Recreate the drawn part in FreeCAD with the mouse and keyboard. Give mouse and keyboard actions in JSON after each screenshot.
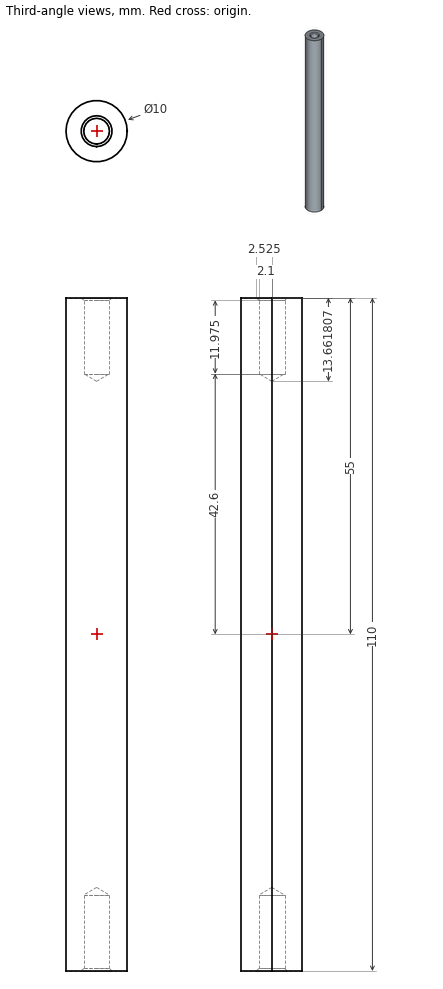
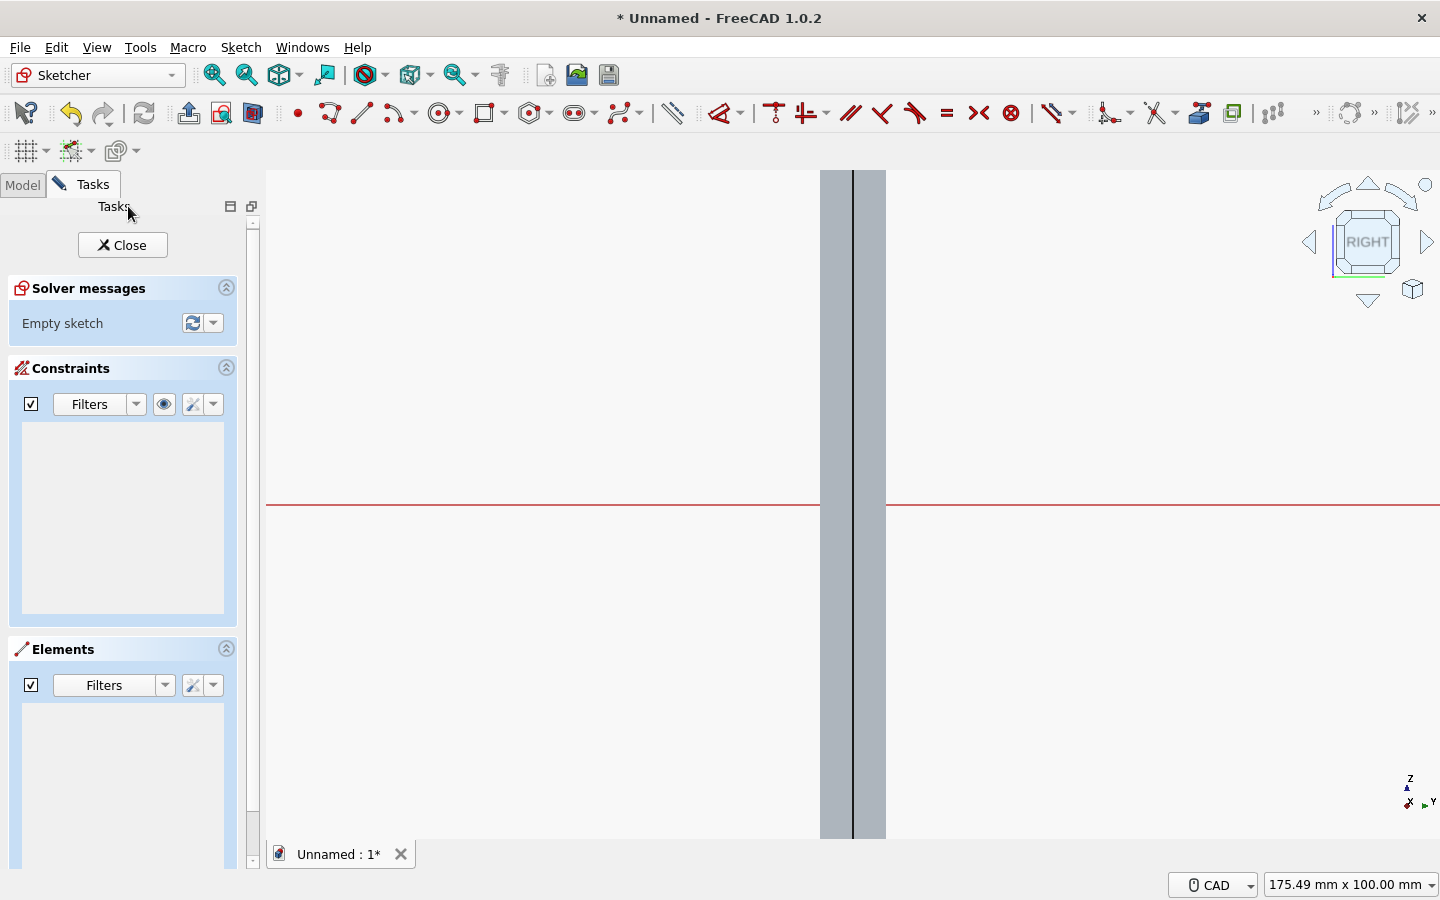
{"action": "left_click", "coordinate": [254, 114]}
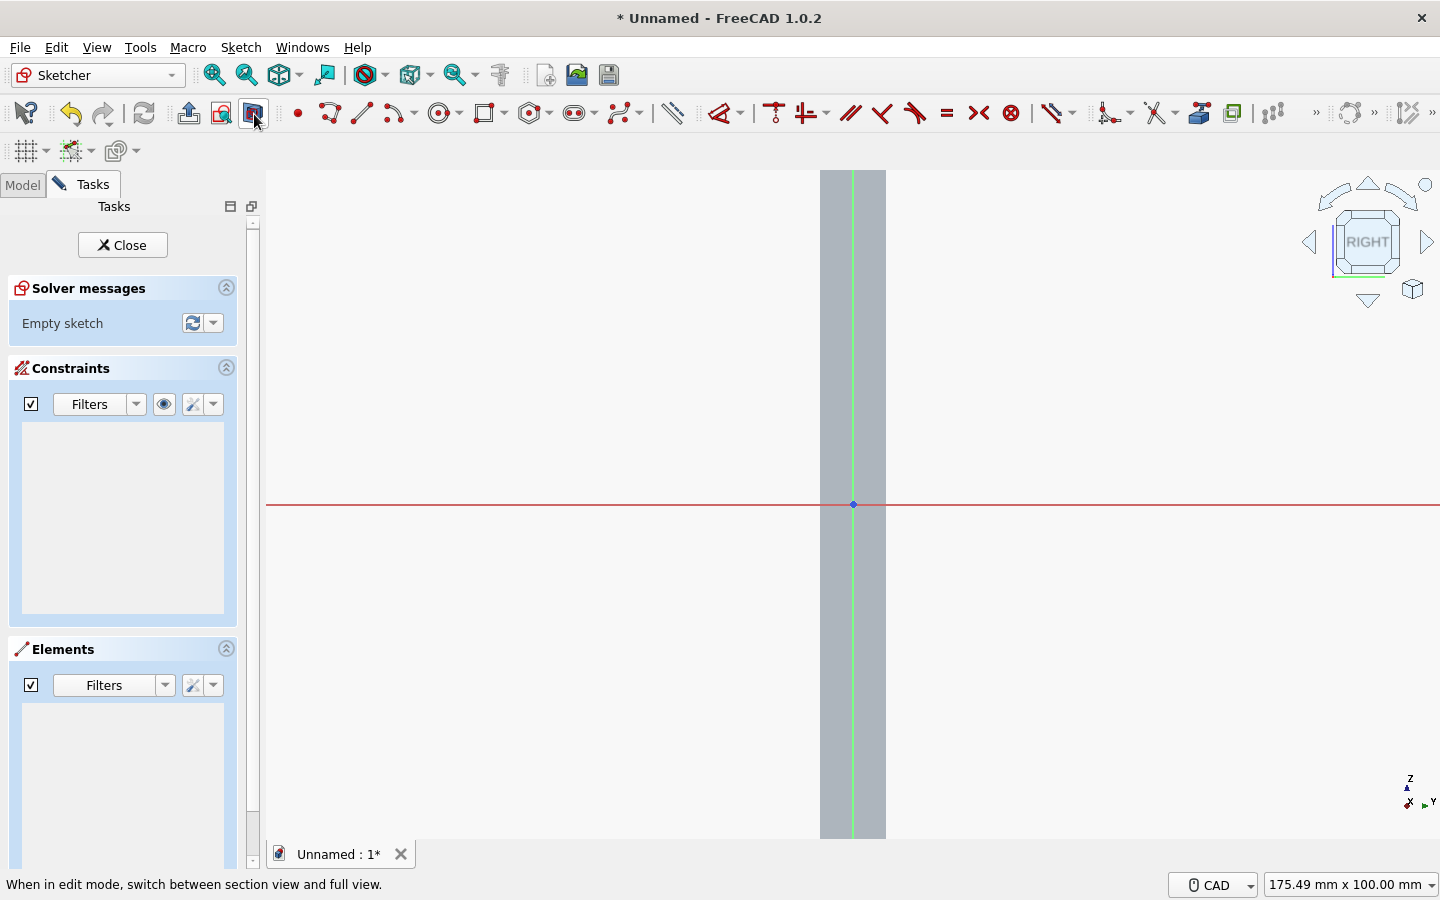
{"action": "scroll", "coordinate": [784, 504], "scroll_direction": "down", "scroll_amount": 5}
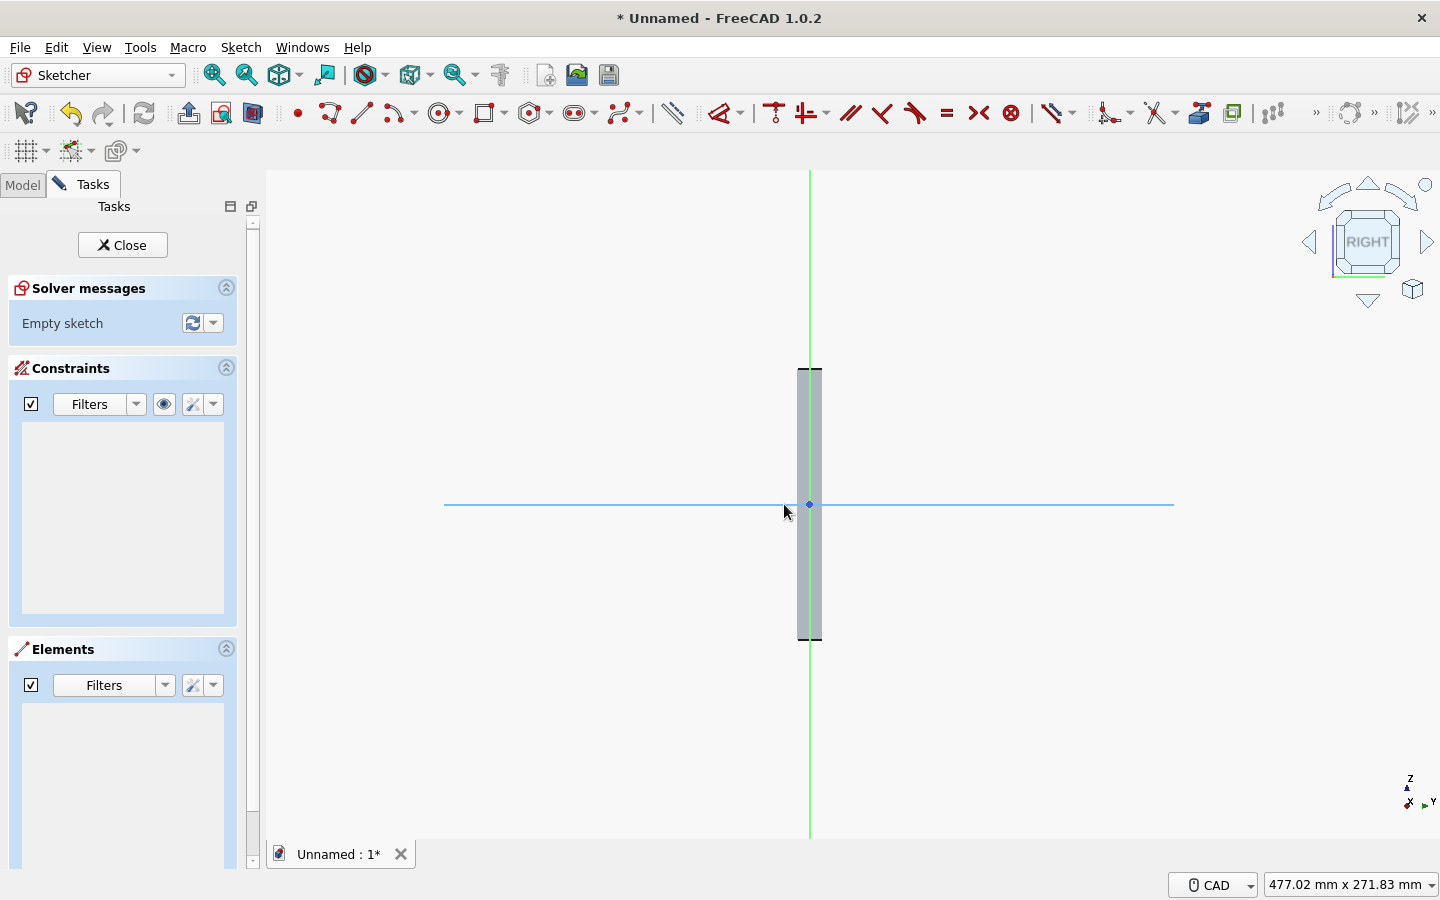
{"action": "scroll", "coordinate": [808, 376], "scroll_direction": "up", "scroll_amount": 13}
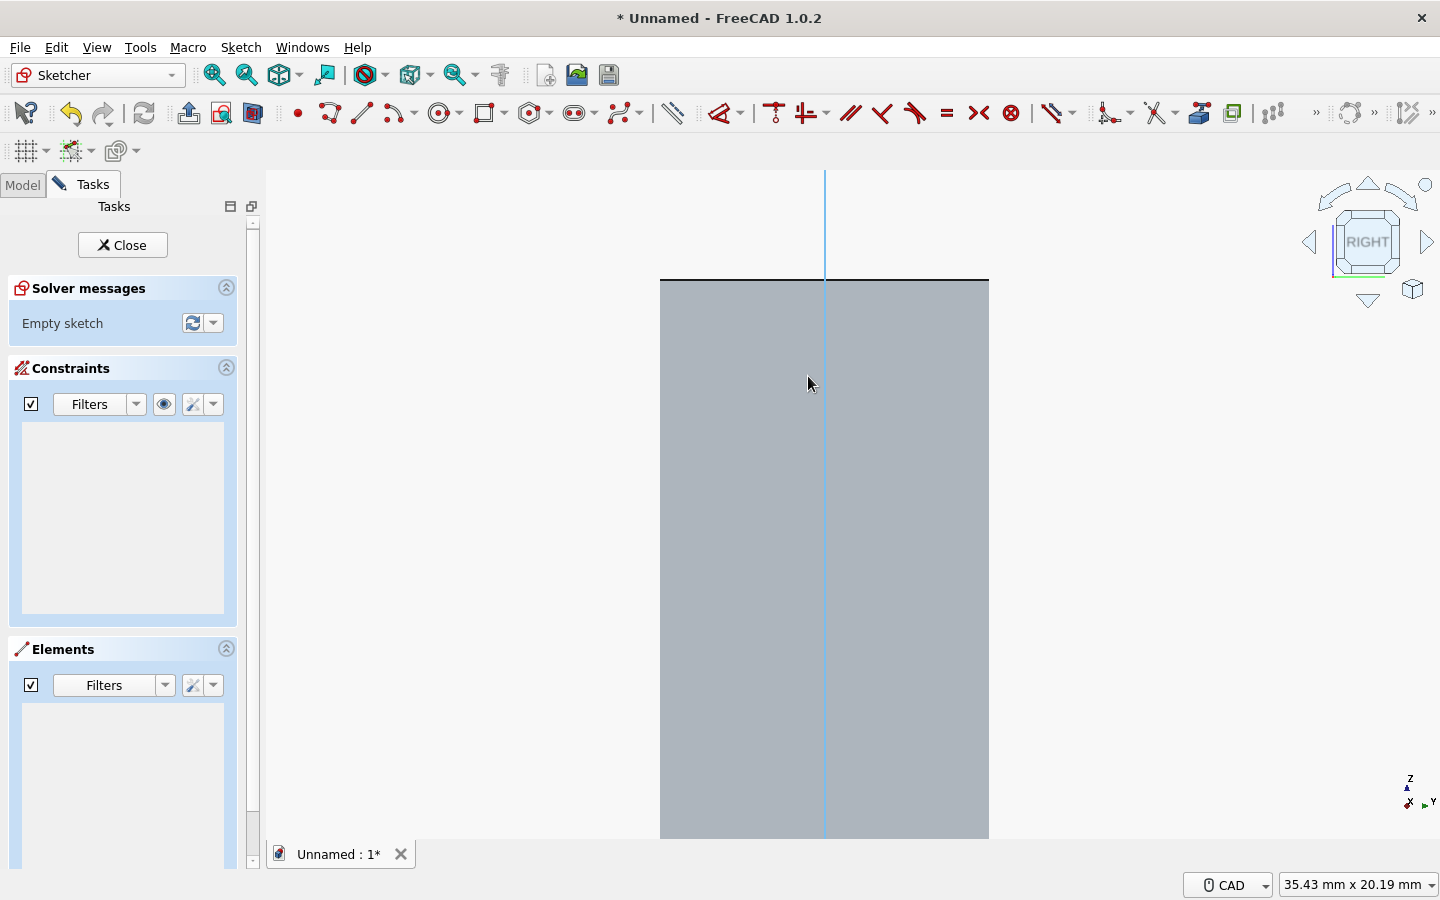
{"action": "left_click", "coordinate": [330, 114]}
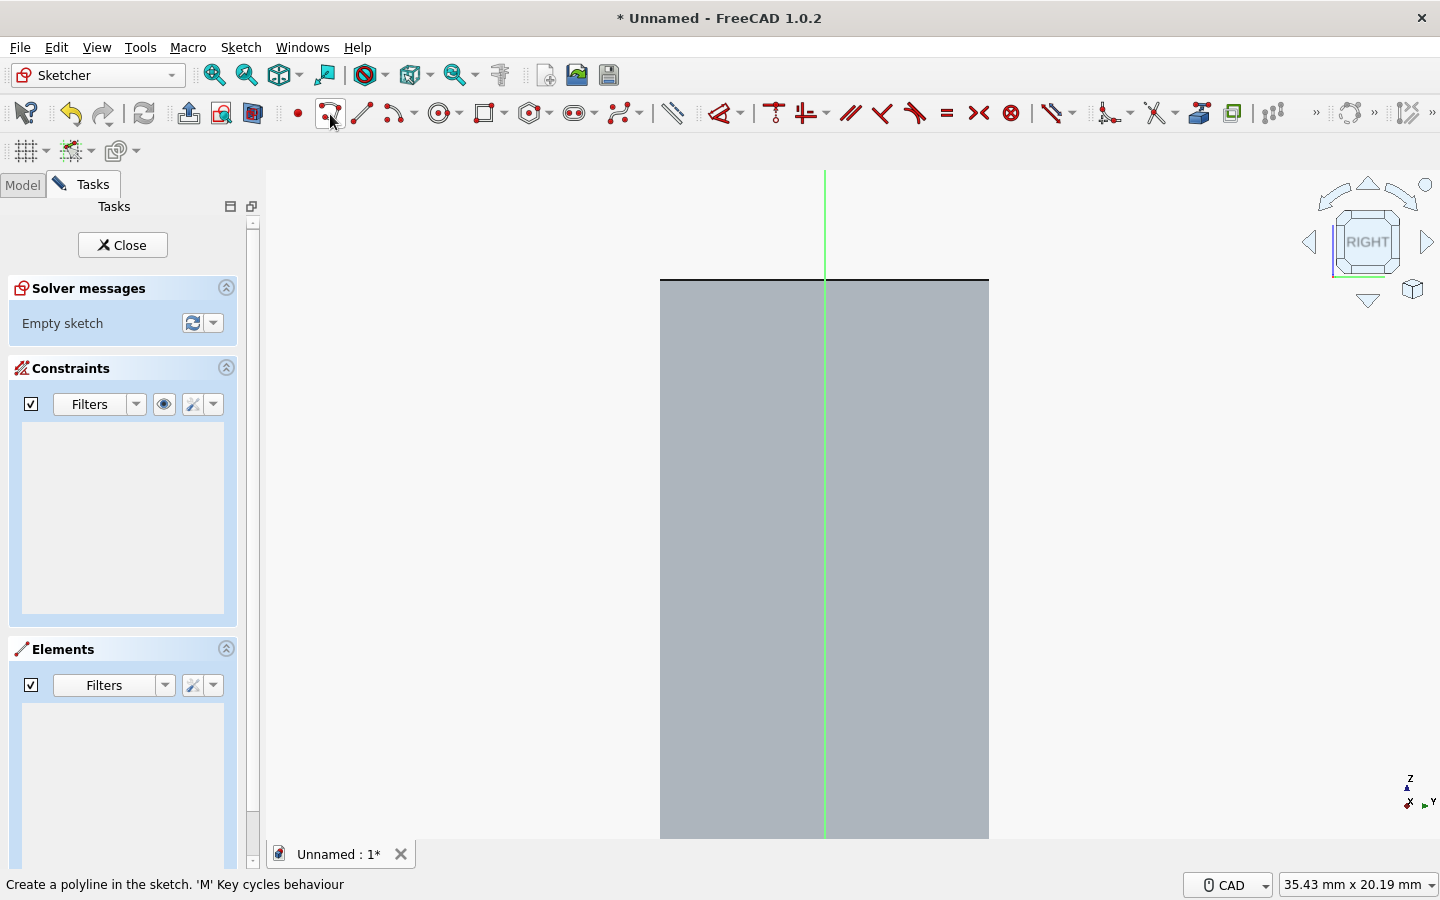
{"action": "left_click", "coordinate": [825, 732]}
{"action": "left_click", "coordinate": [816, 280]}
{"action": "left_click", "coordinate": [741, 280]}
{"action": "left_click", "coordinate": [755, 294]}
{"action": "left_click", "coordinate": [755, 691]}
{"action": "left_click", "coordinate": [825, 733]}
{"action": "key", "text": "Escape"}
{"action": "key", "text": "Escape"}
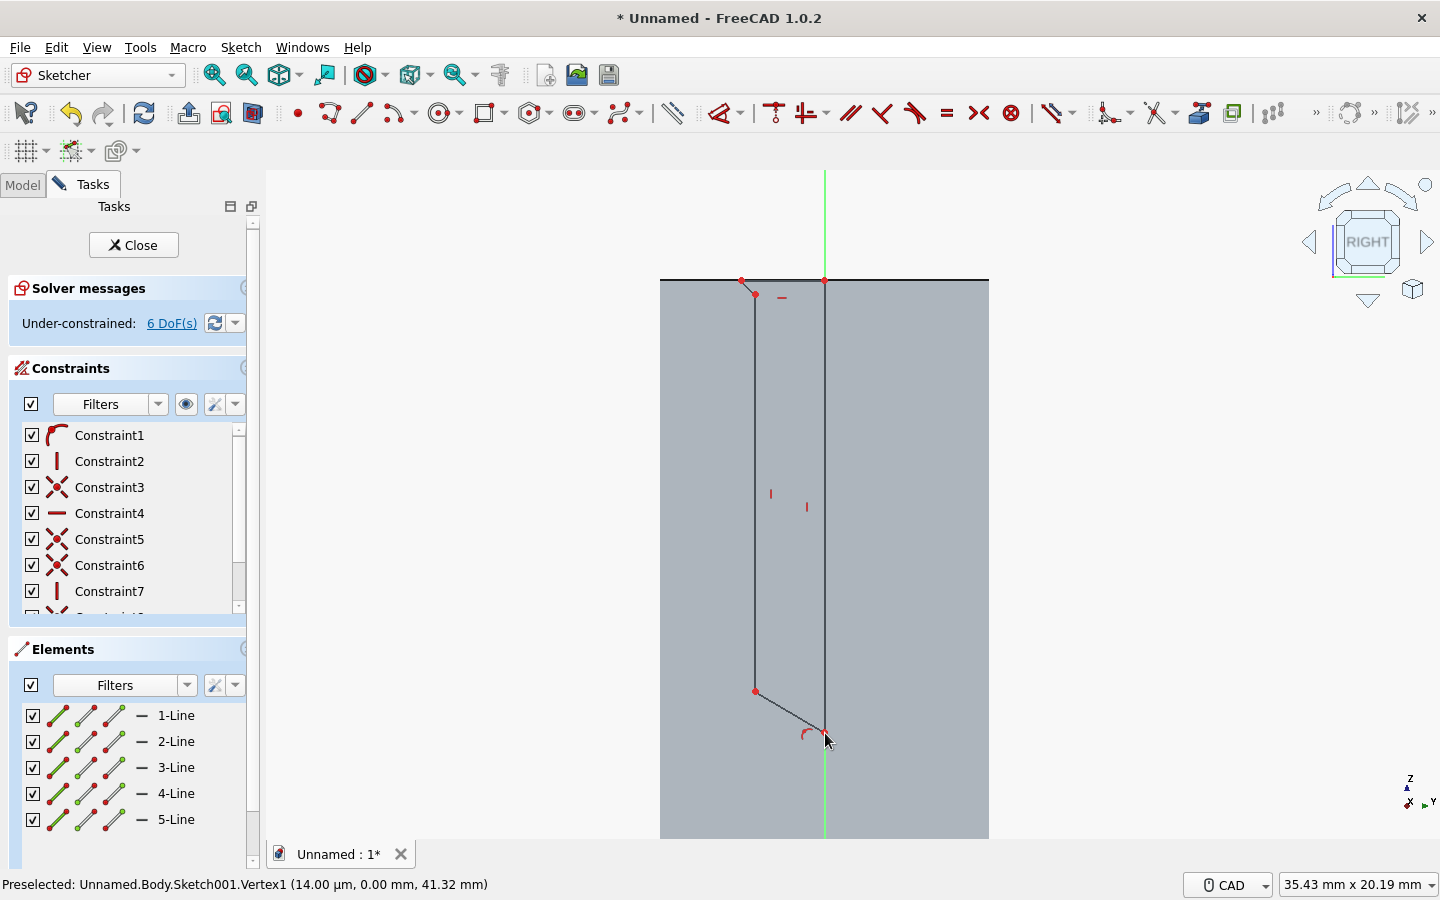
{"action": "left_click", "coordinate": [720, 114]}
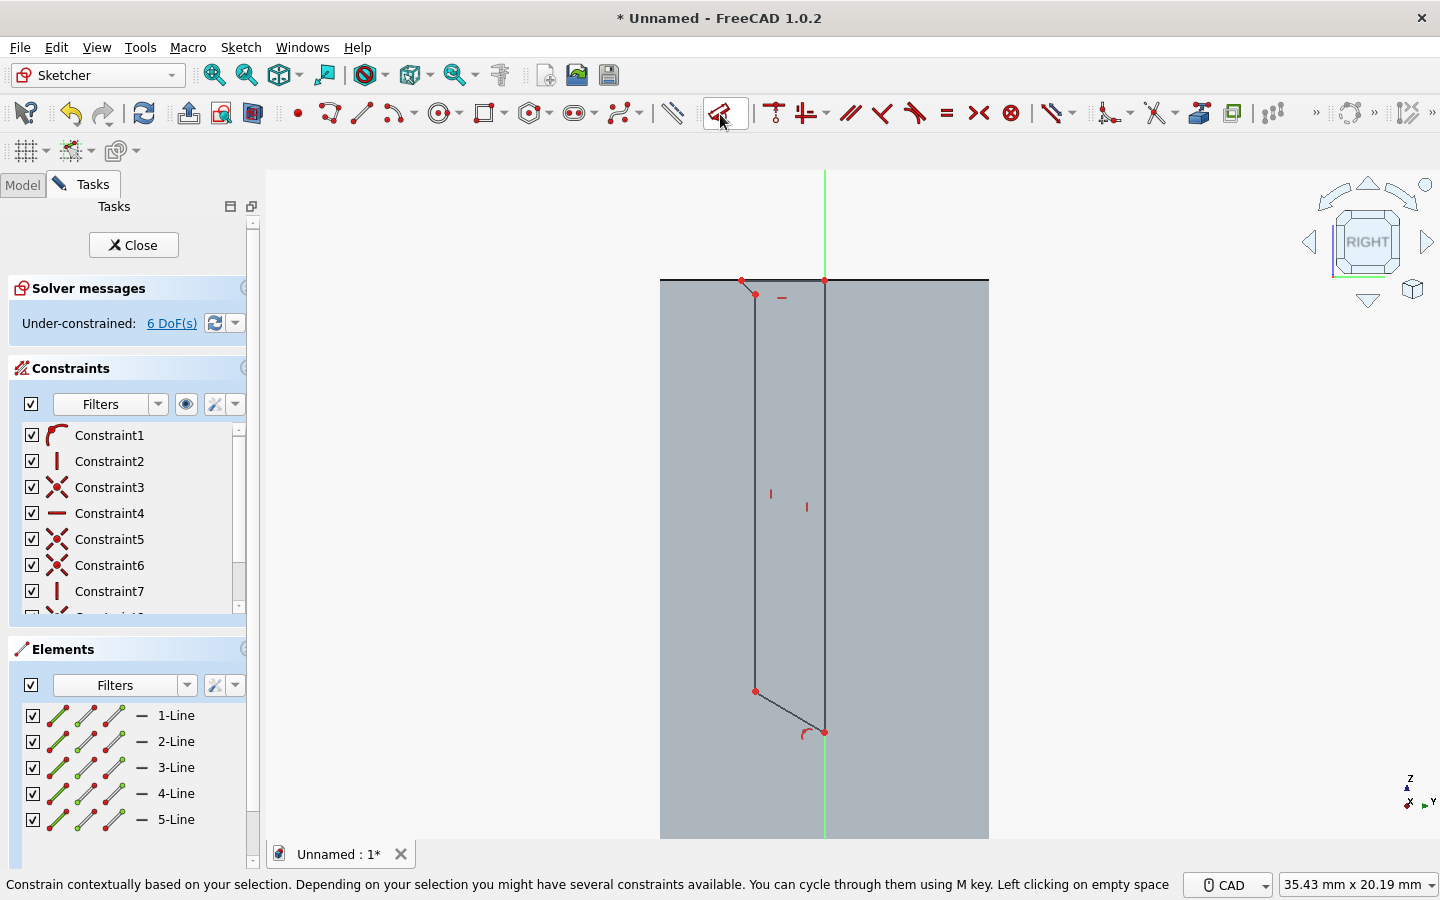
{"action": "left_click", "coordinate": [825, 281]}
{"action": "left_click", "coordinate": [859, 546]}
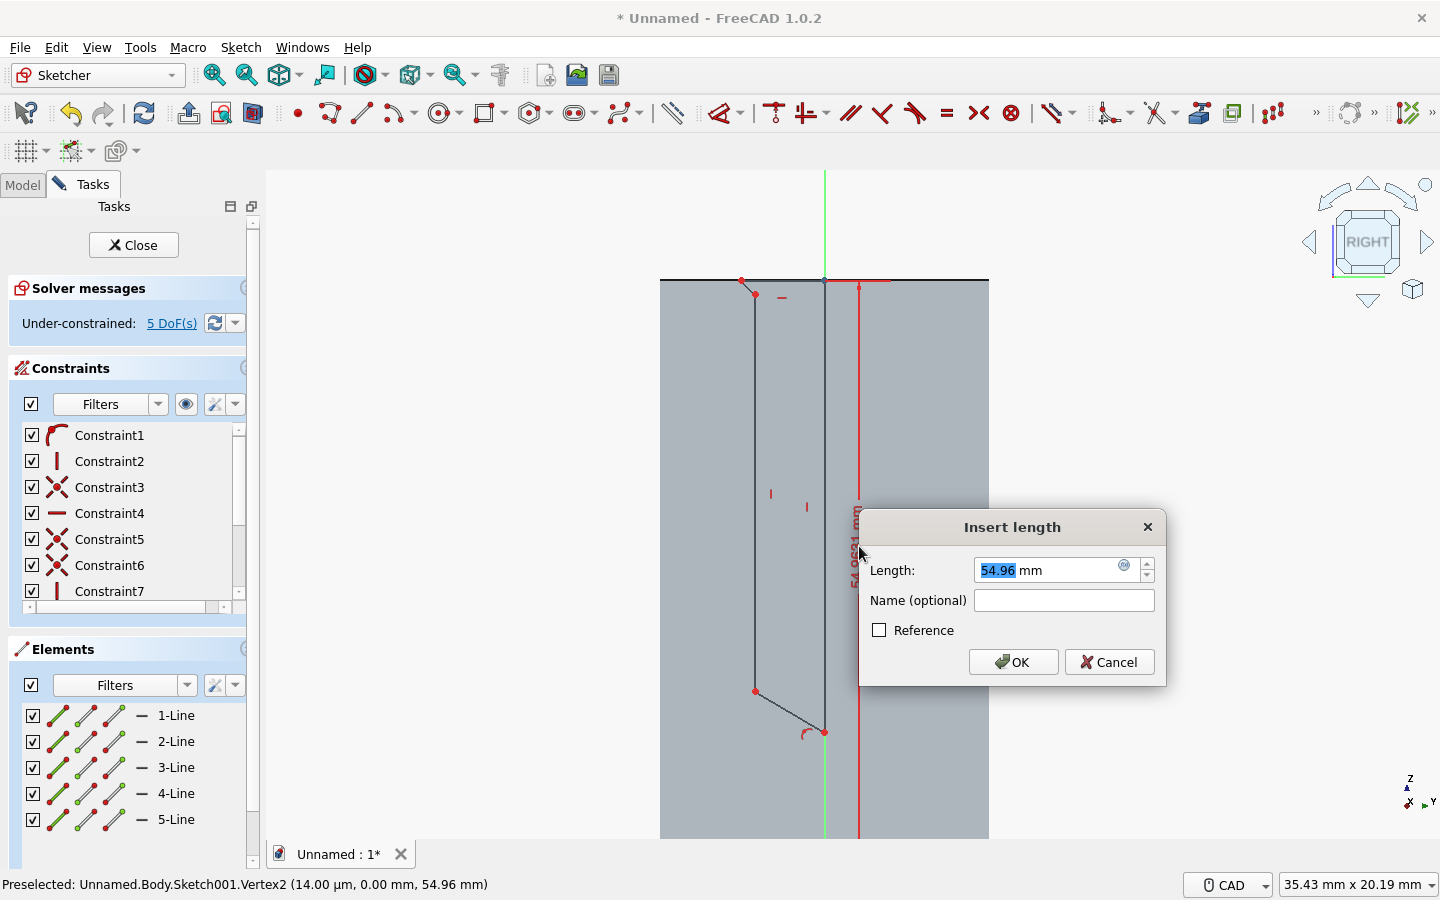
{"action": "type", "text": "55"}
{"action": "key", "text": "Return"}